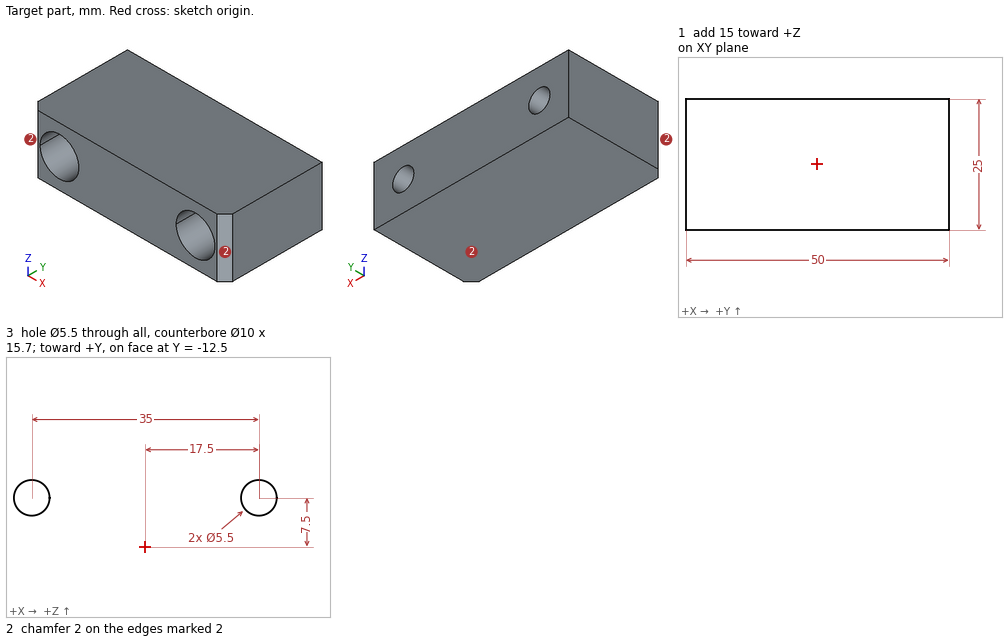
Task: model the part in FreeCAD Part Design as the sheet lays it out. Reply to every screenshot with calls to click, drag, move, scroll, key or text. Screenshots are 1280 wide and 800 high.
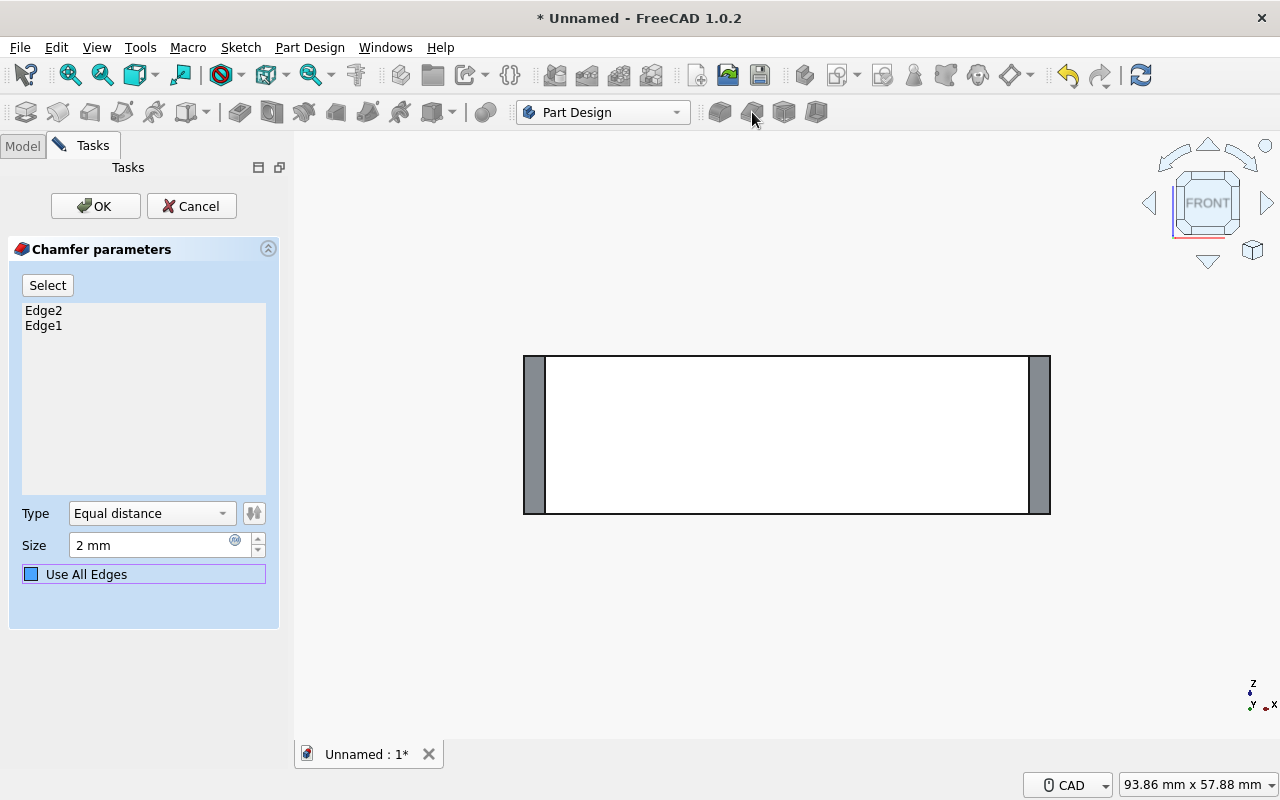
click(96, 206)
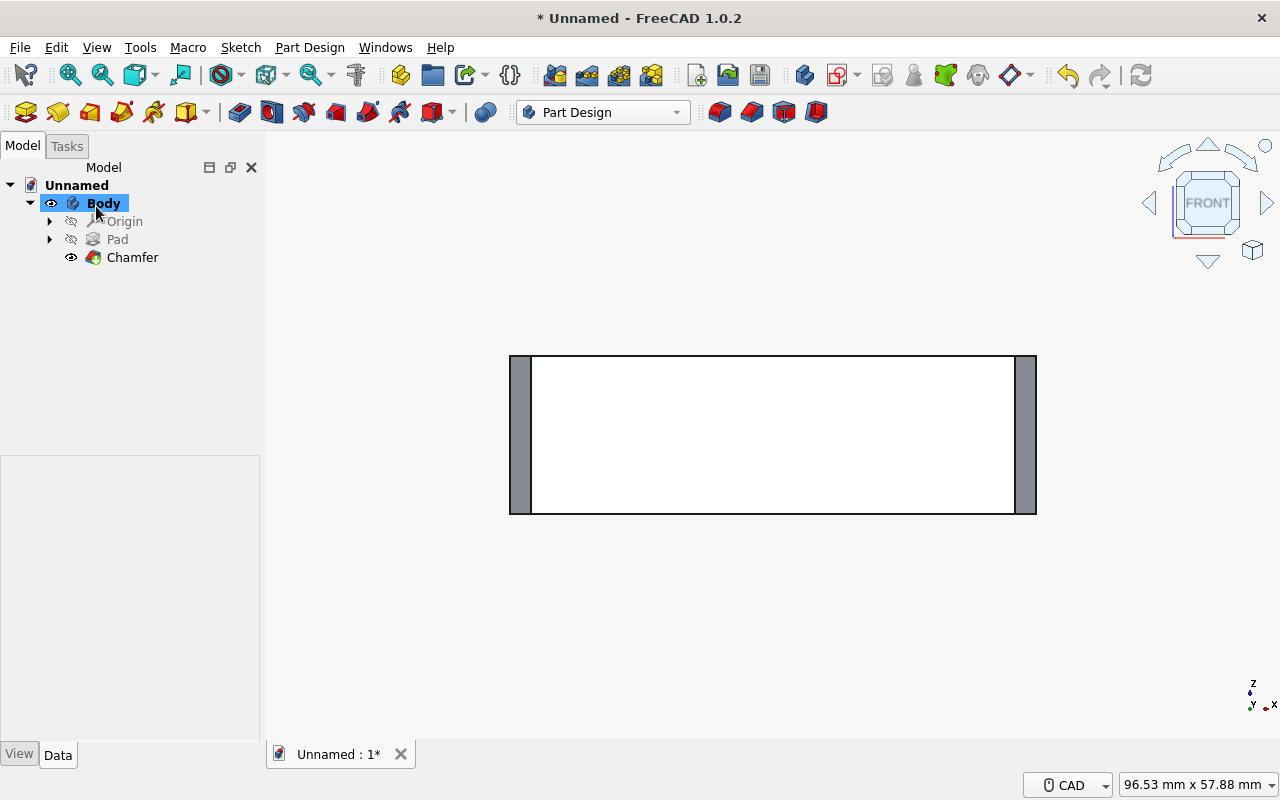
click(911, 434)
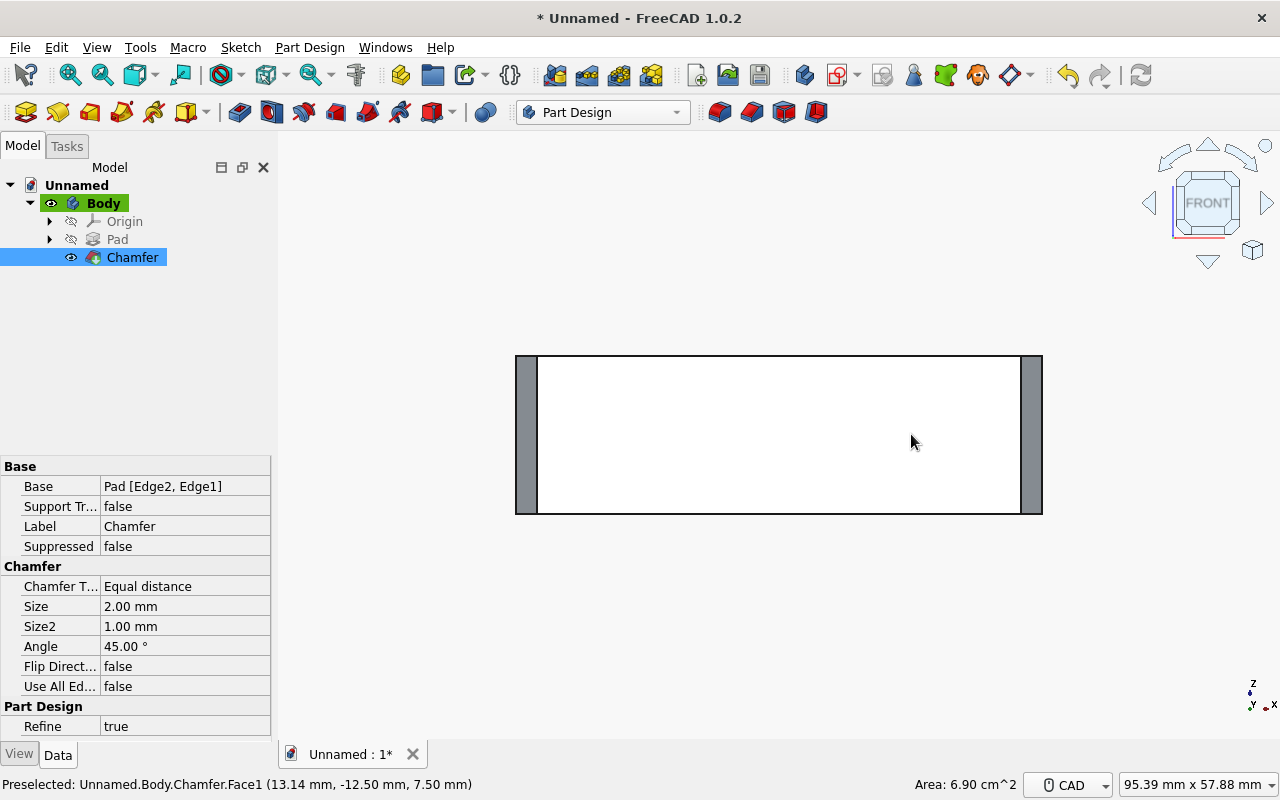
click(838, 76)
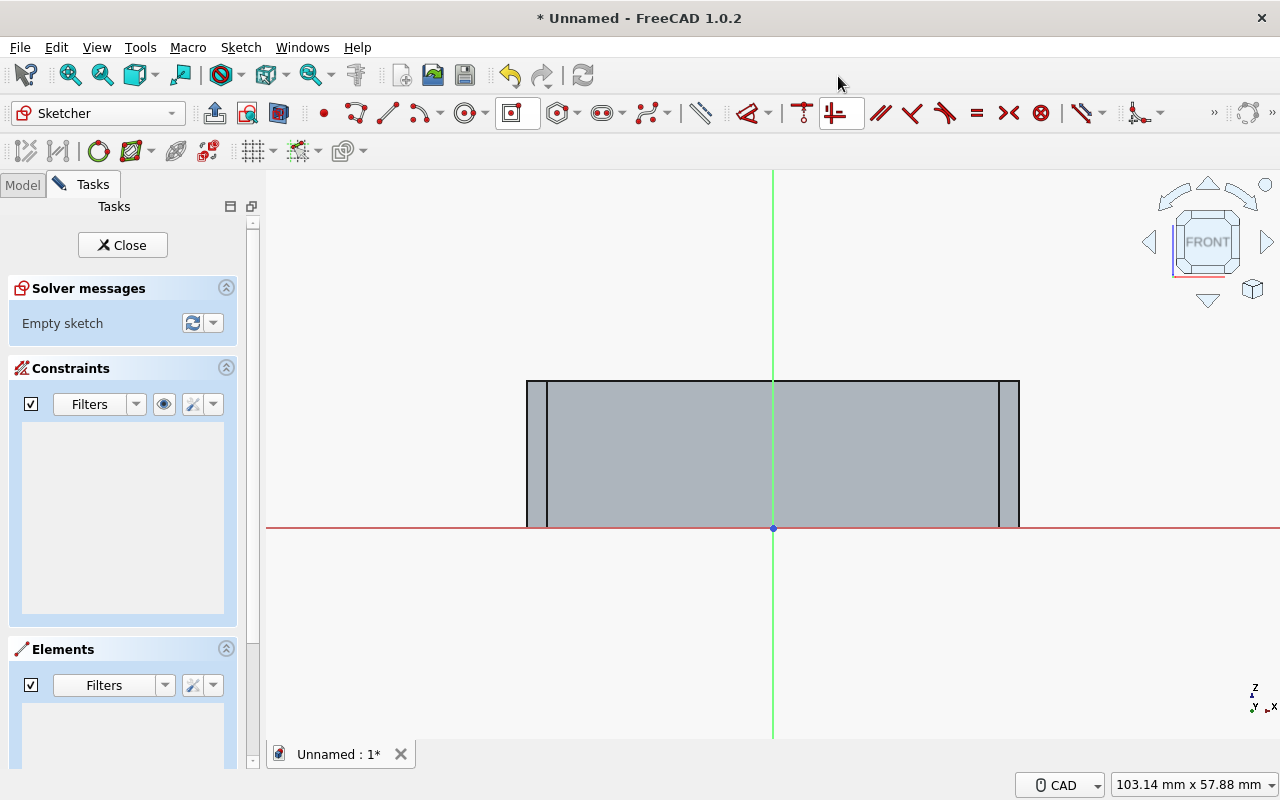
scroll(912, 525, up, 2)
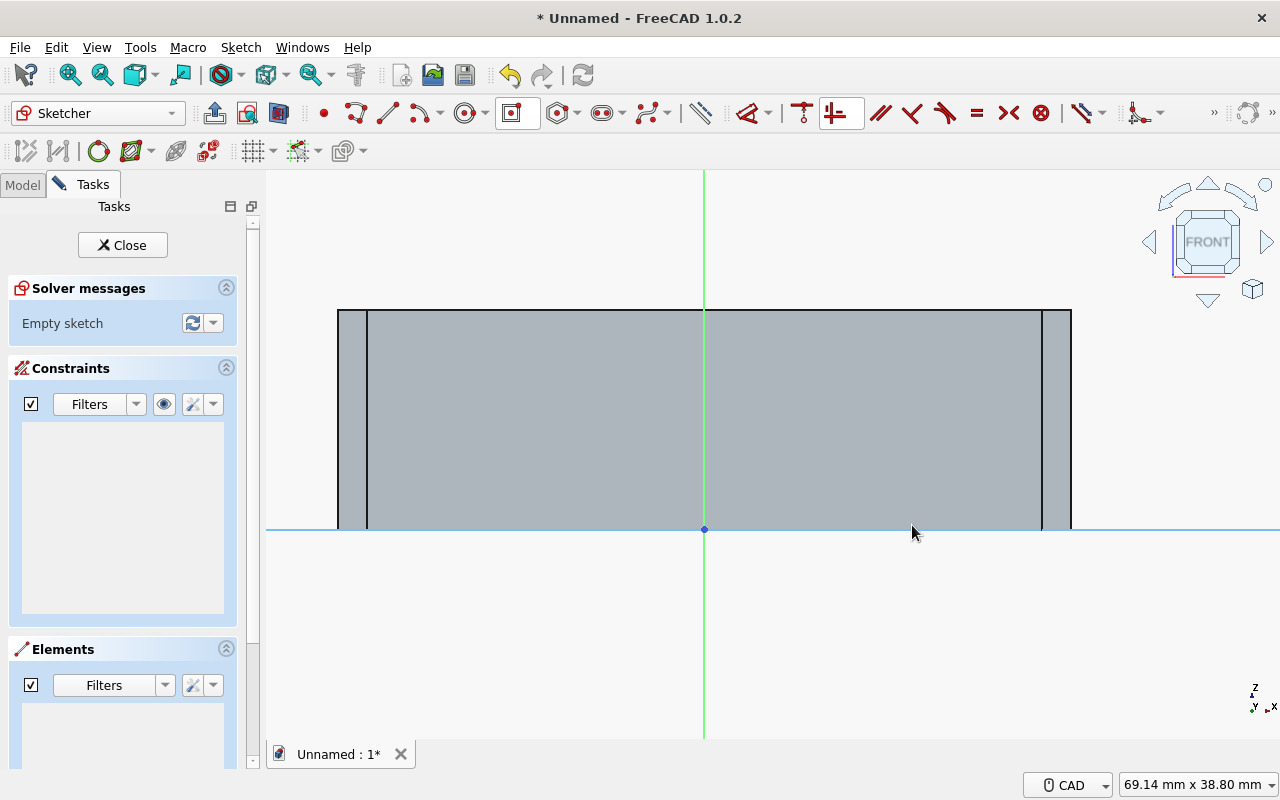
click(466, 114)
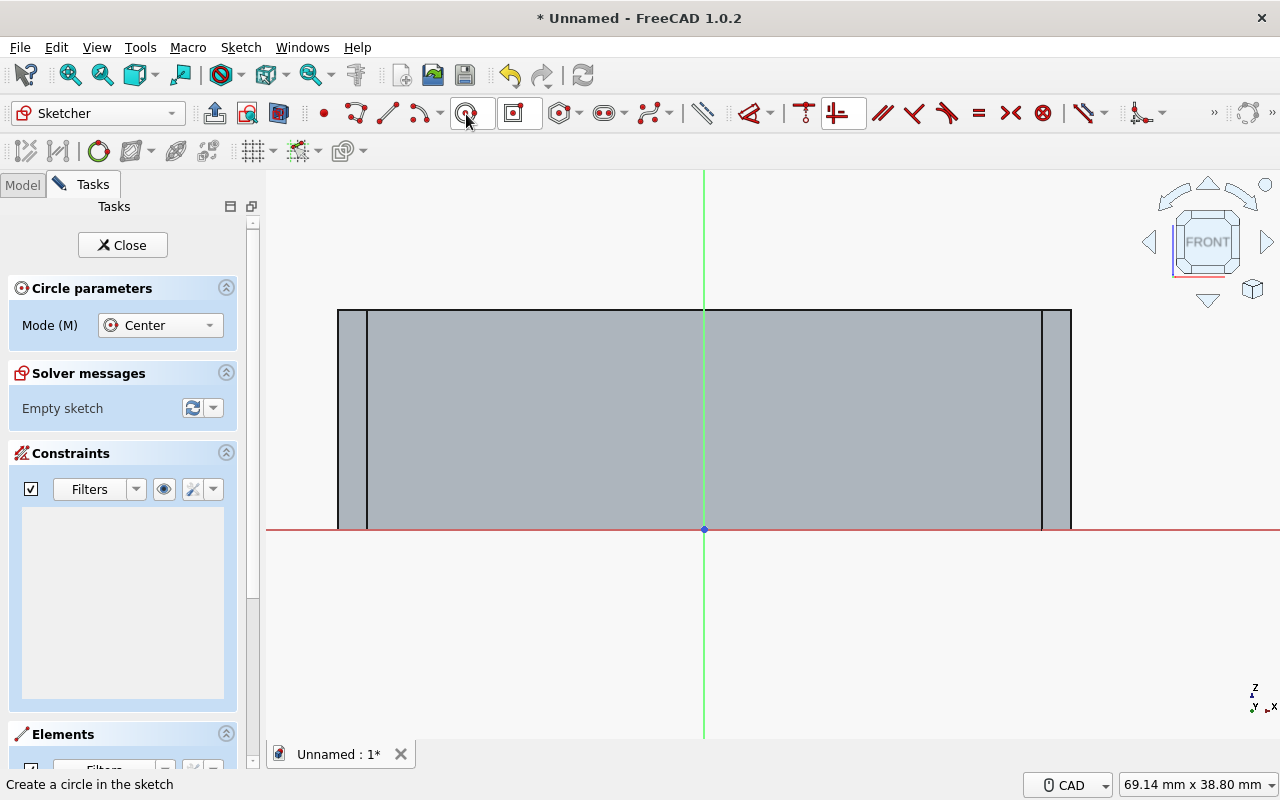
click(961, 420)
move(989, 391)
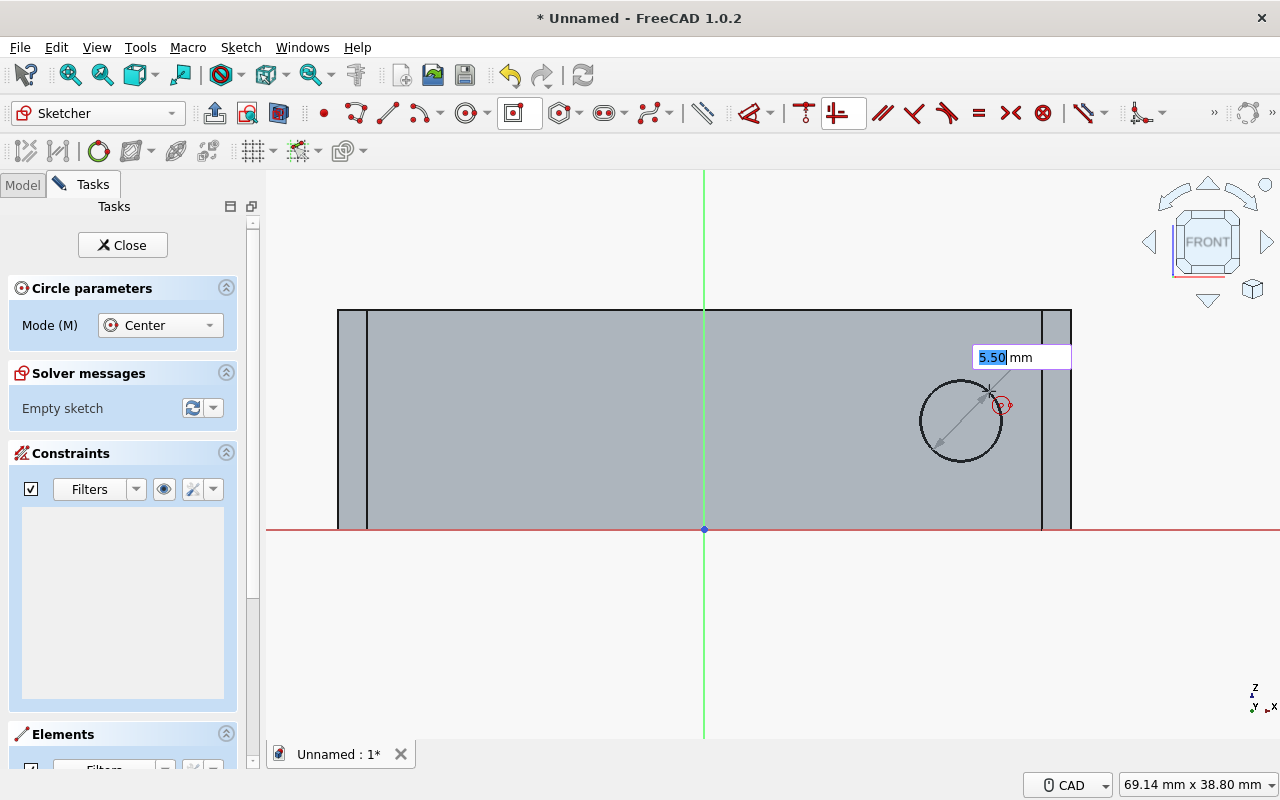
text(5.5)
key(Return)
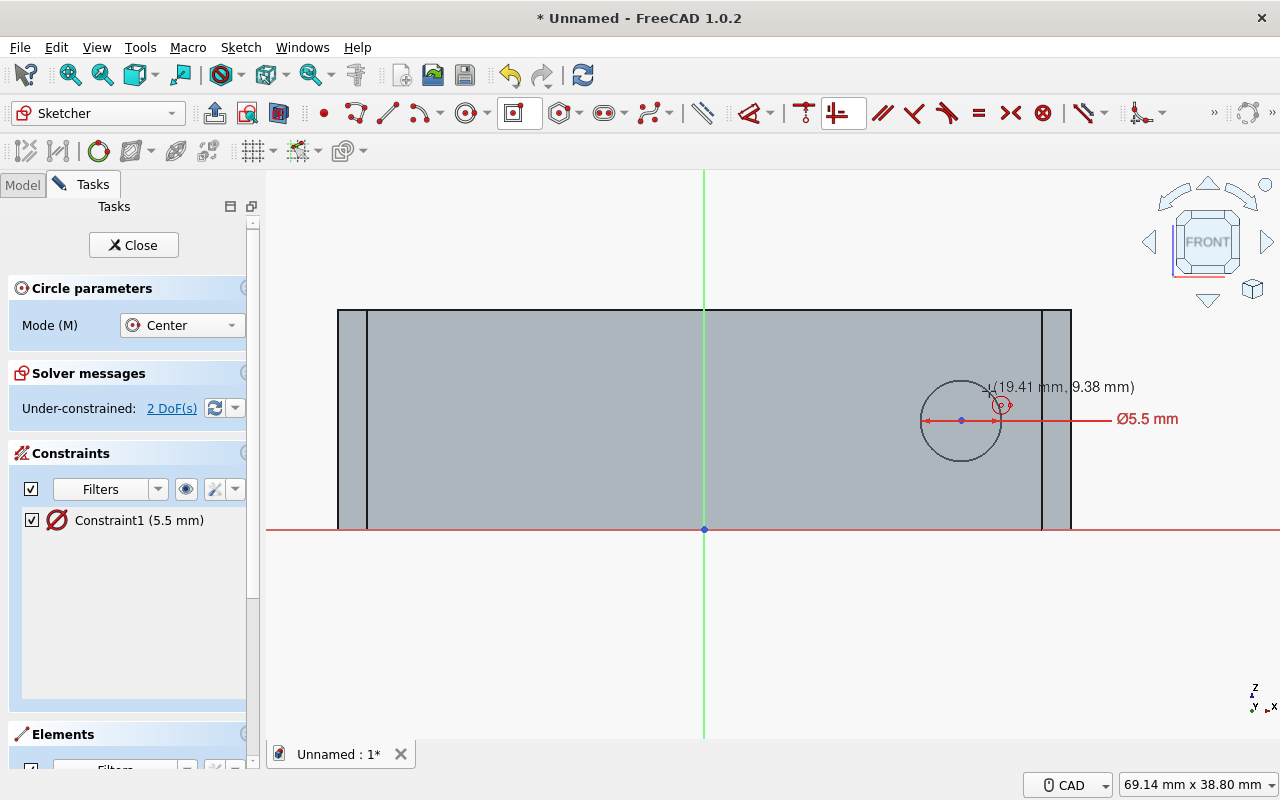
click(448, 420)
move(476, 391)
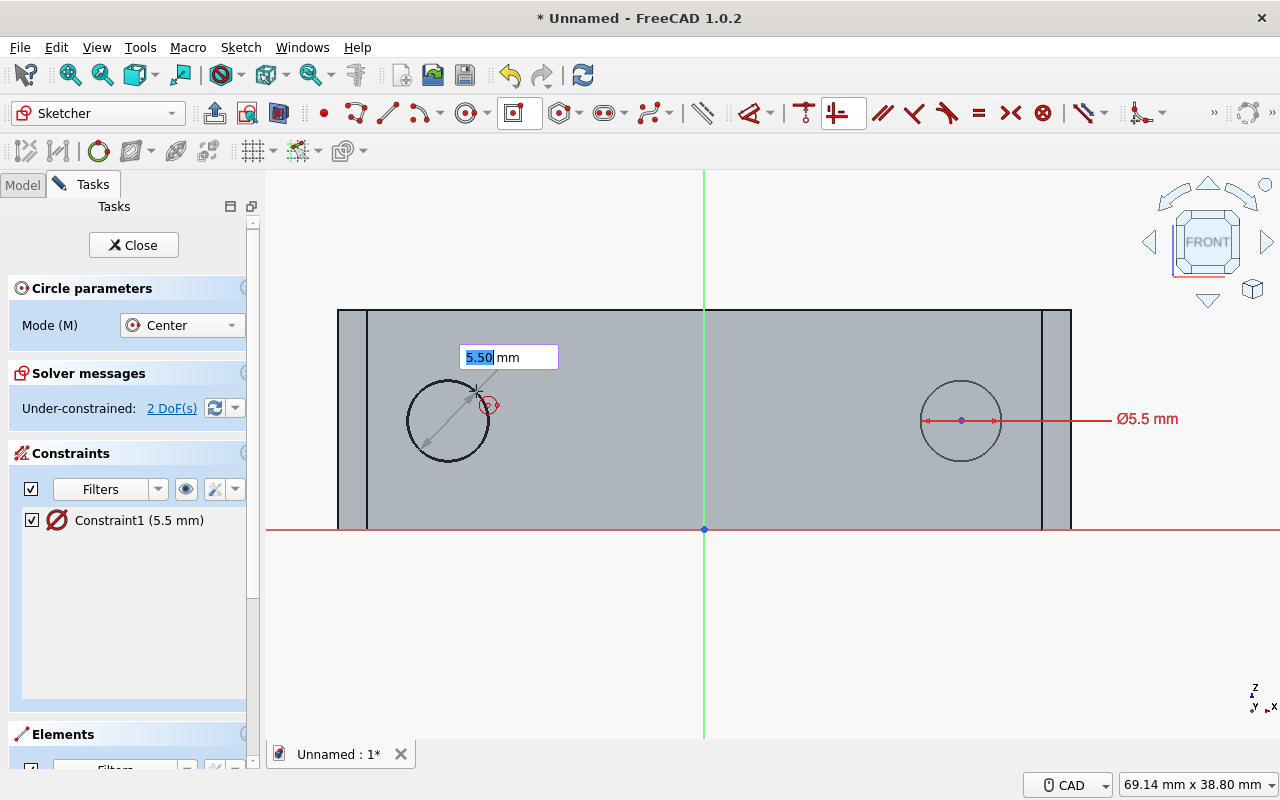
text(5.5)
key(Return)
key(Escape)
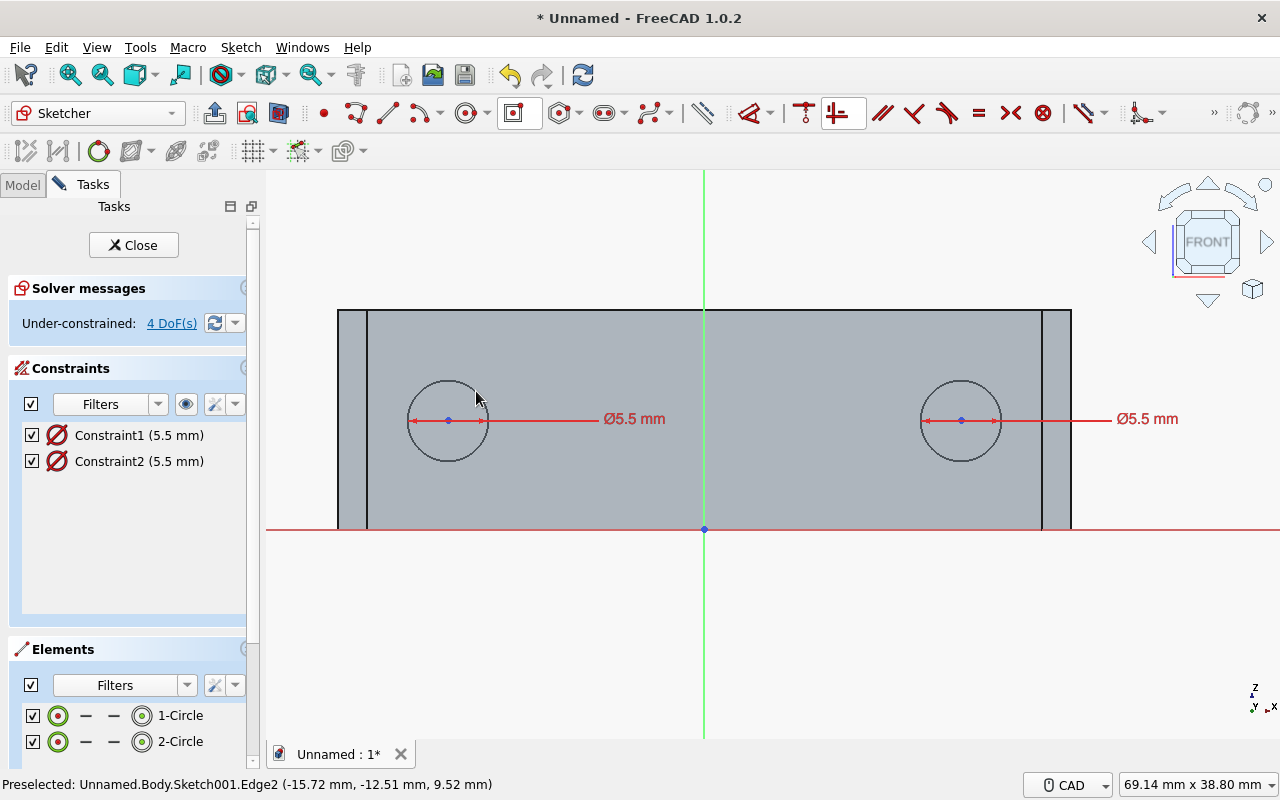
click(961, 421)